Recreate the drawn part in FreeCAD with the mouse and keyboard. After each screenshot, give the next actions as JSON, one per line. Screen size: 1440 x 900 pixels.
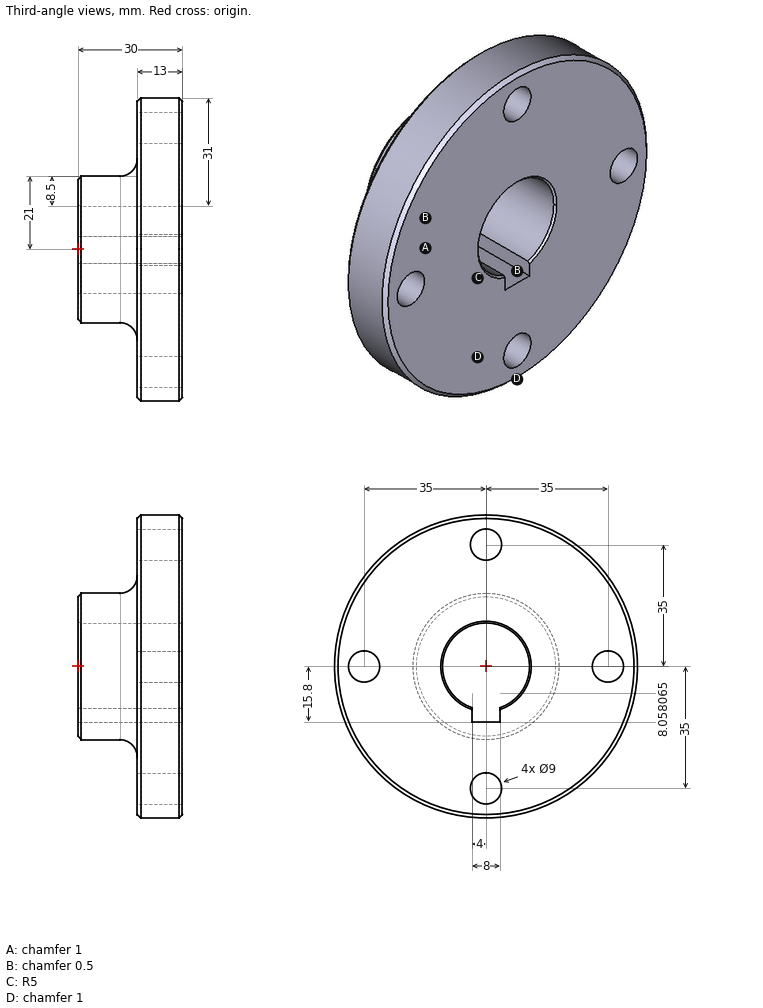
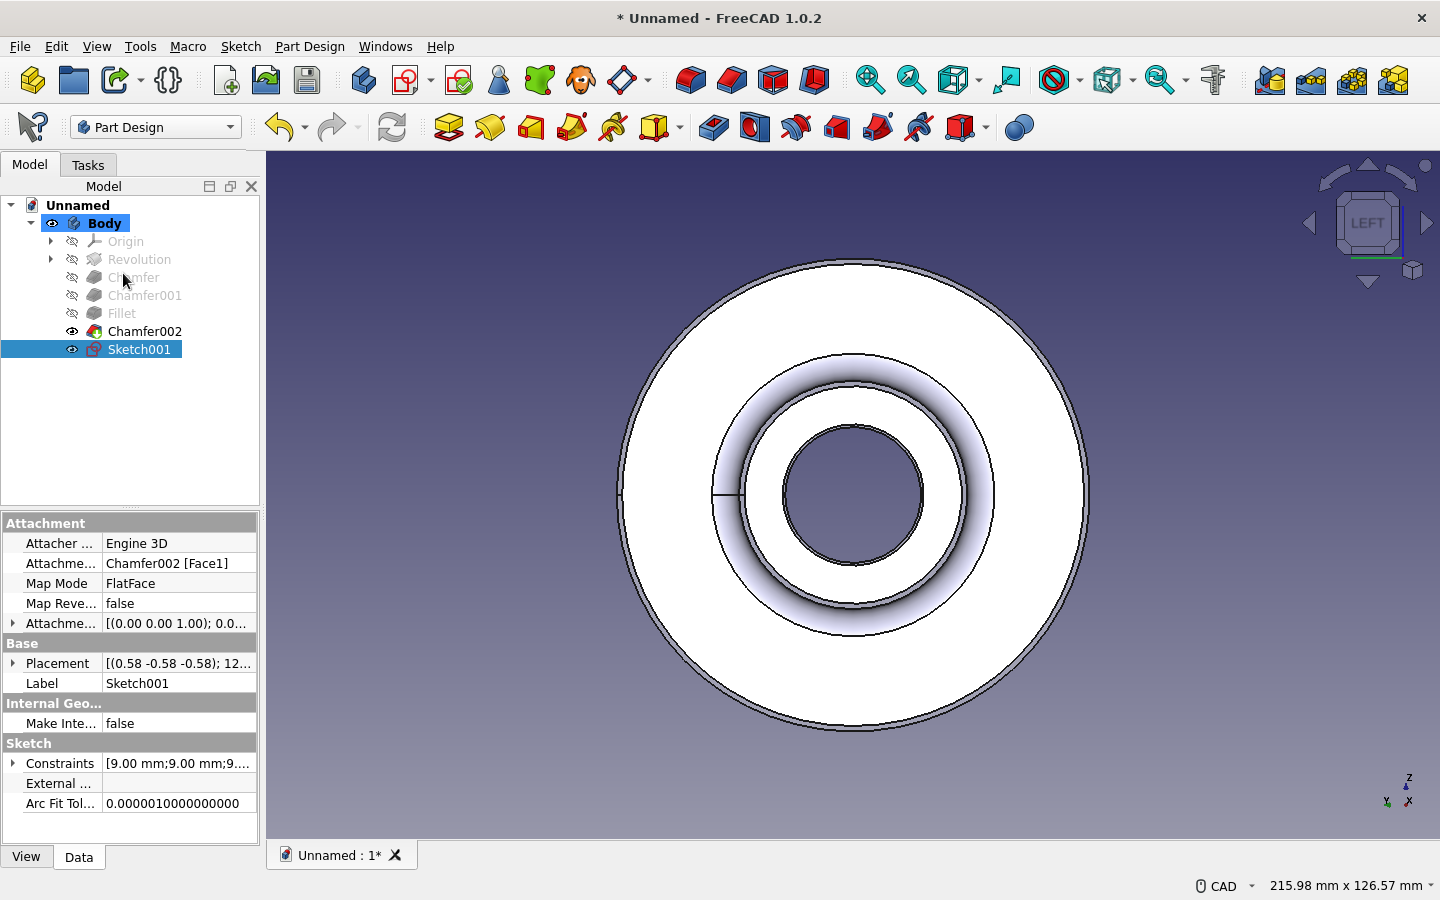
{"action": "left_click", "coordinate": [714, 128]}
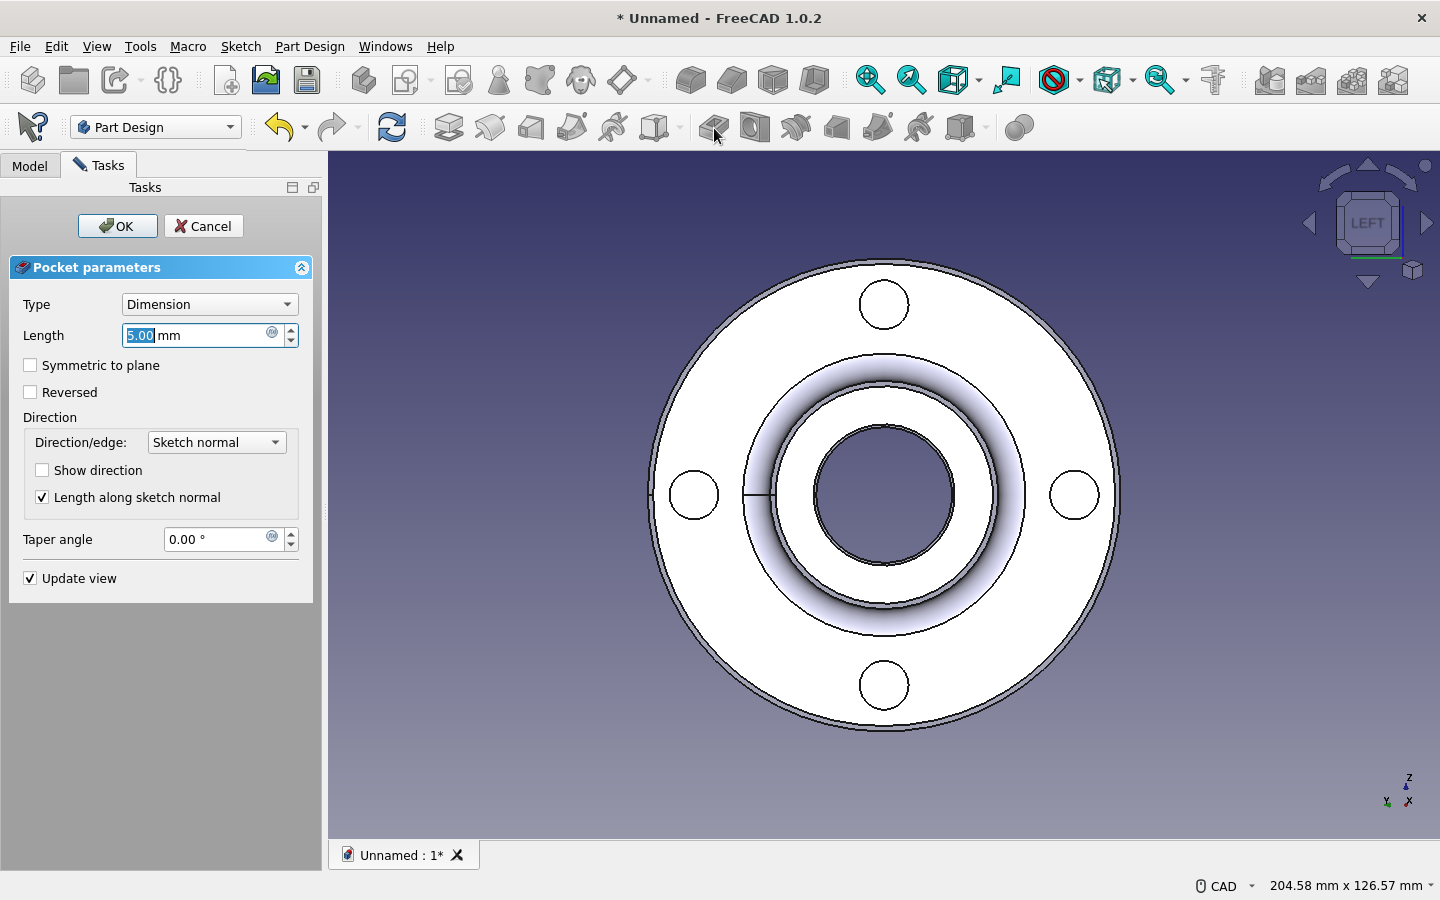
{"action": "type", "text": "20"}
{"action": "key", "text": "Tab"}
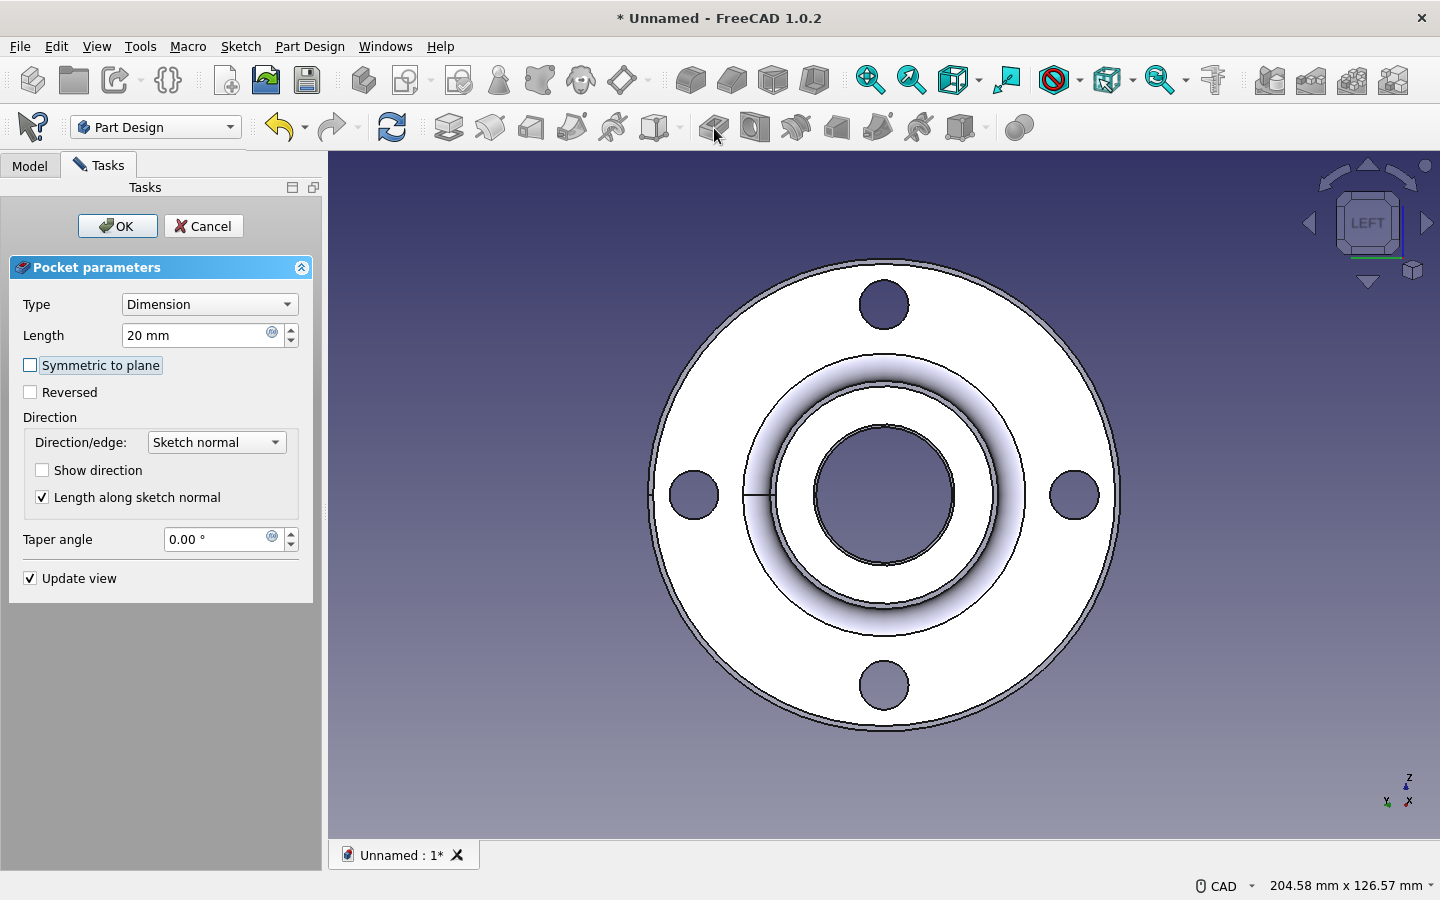
{"action": "left_click", "coordinate": [118, 226]}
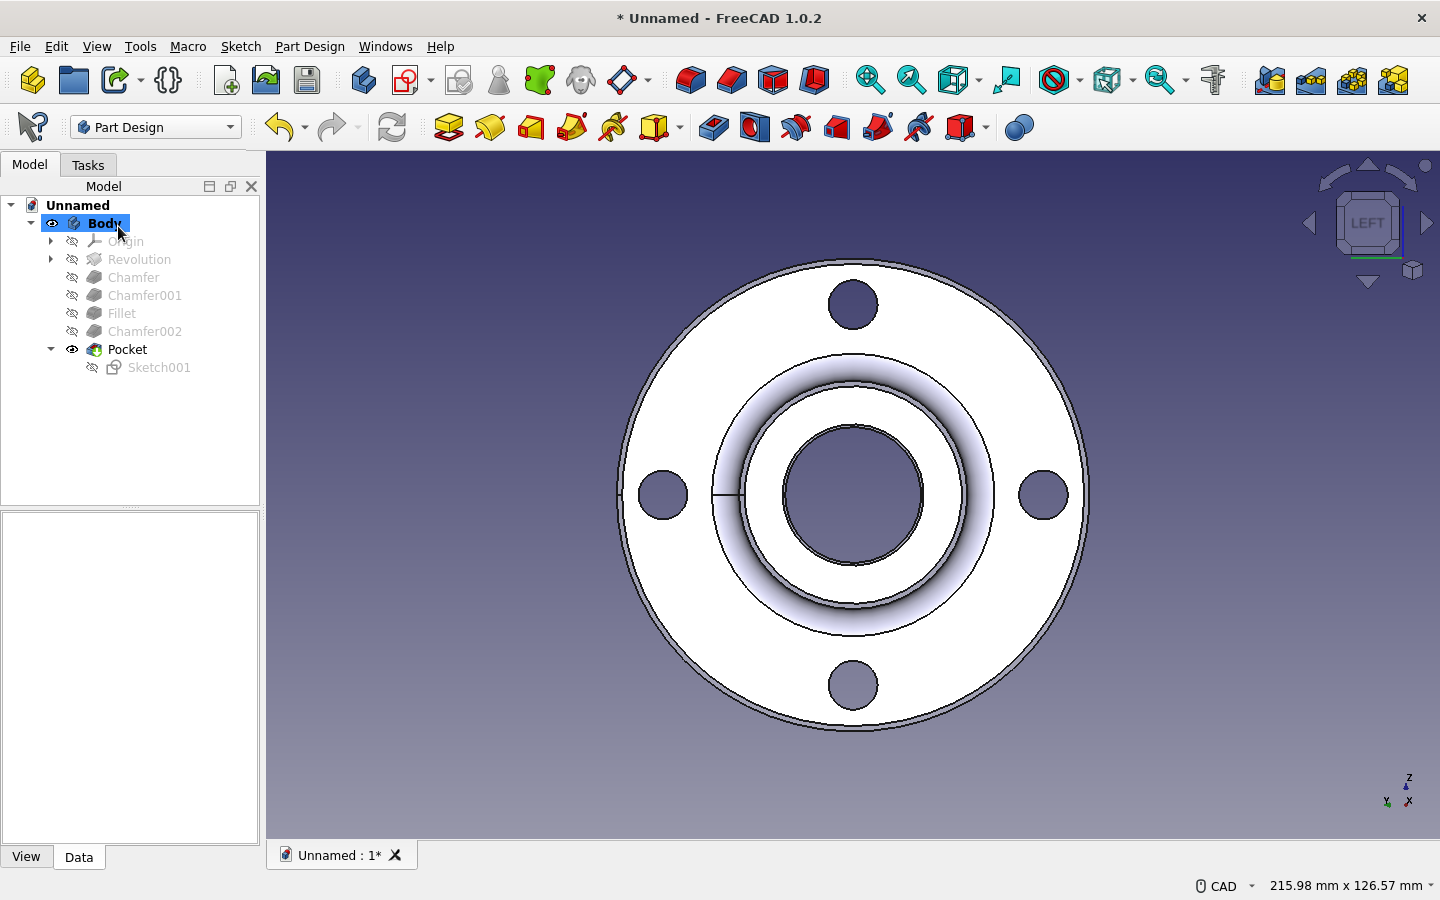
{"action": "key", "text": "0"}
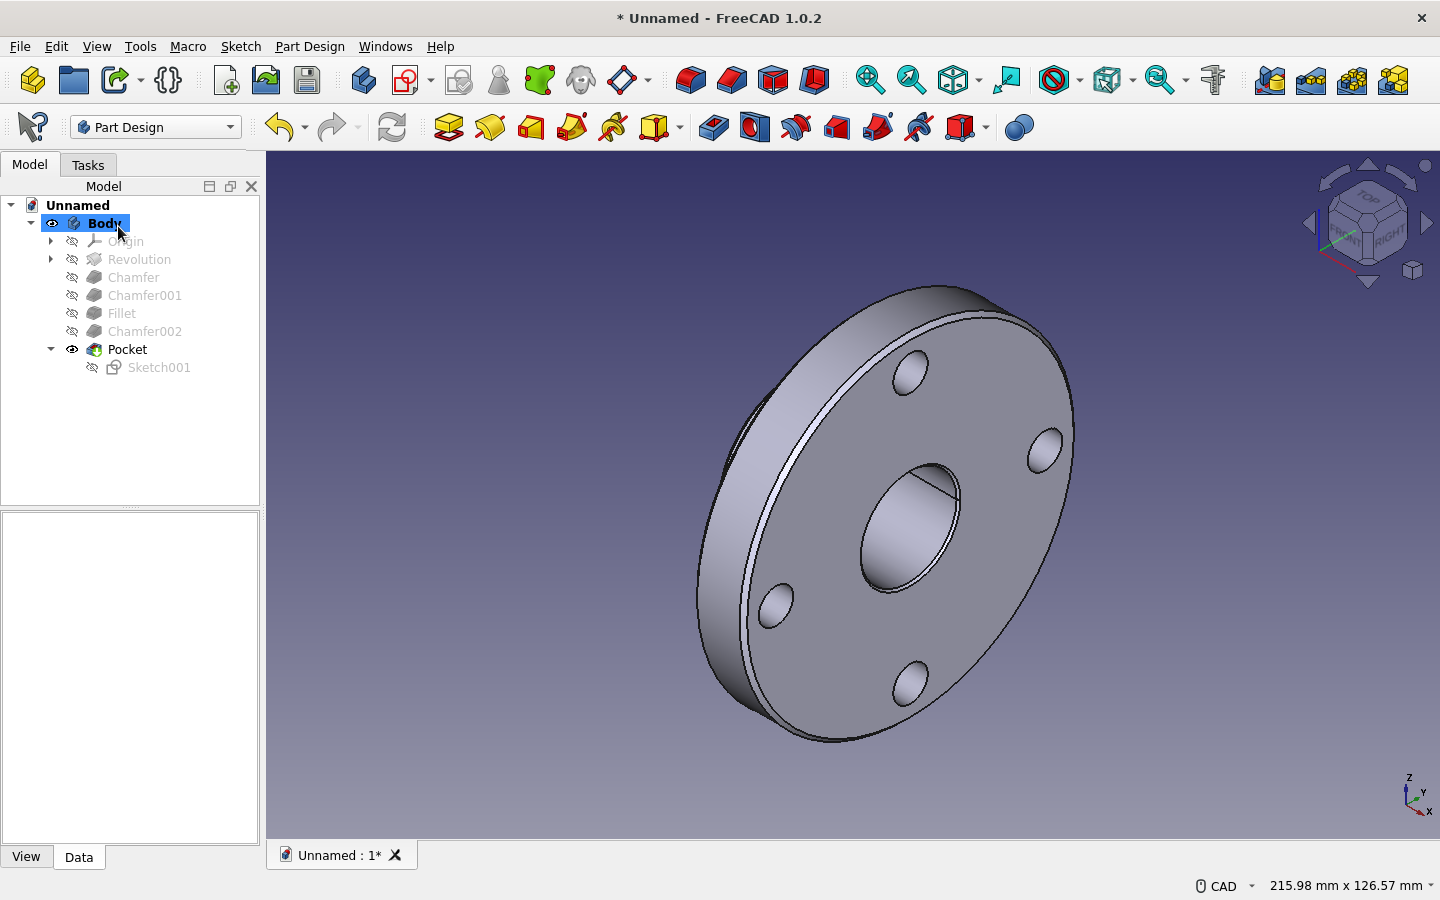
{"action": "left_click", "coordinate": [1004, 420]}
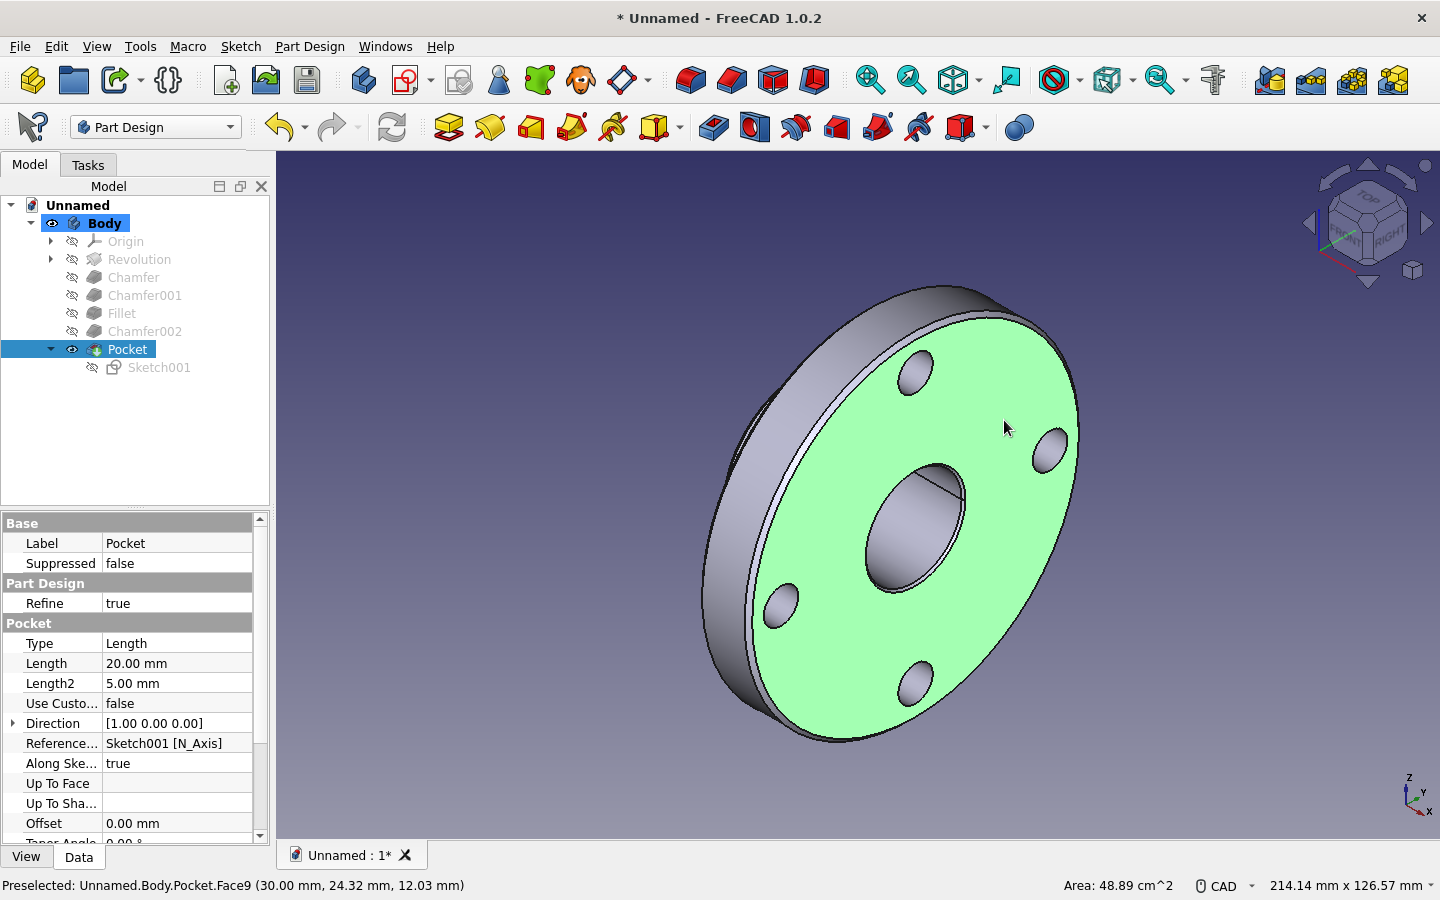
{"action": "left_click", "coordinate": [404, 80]}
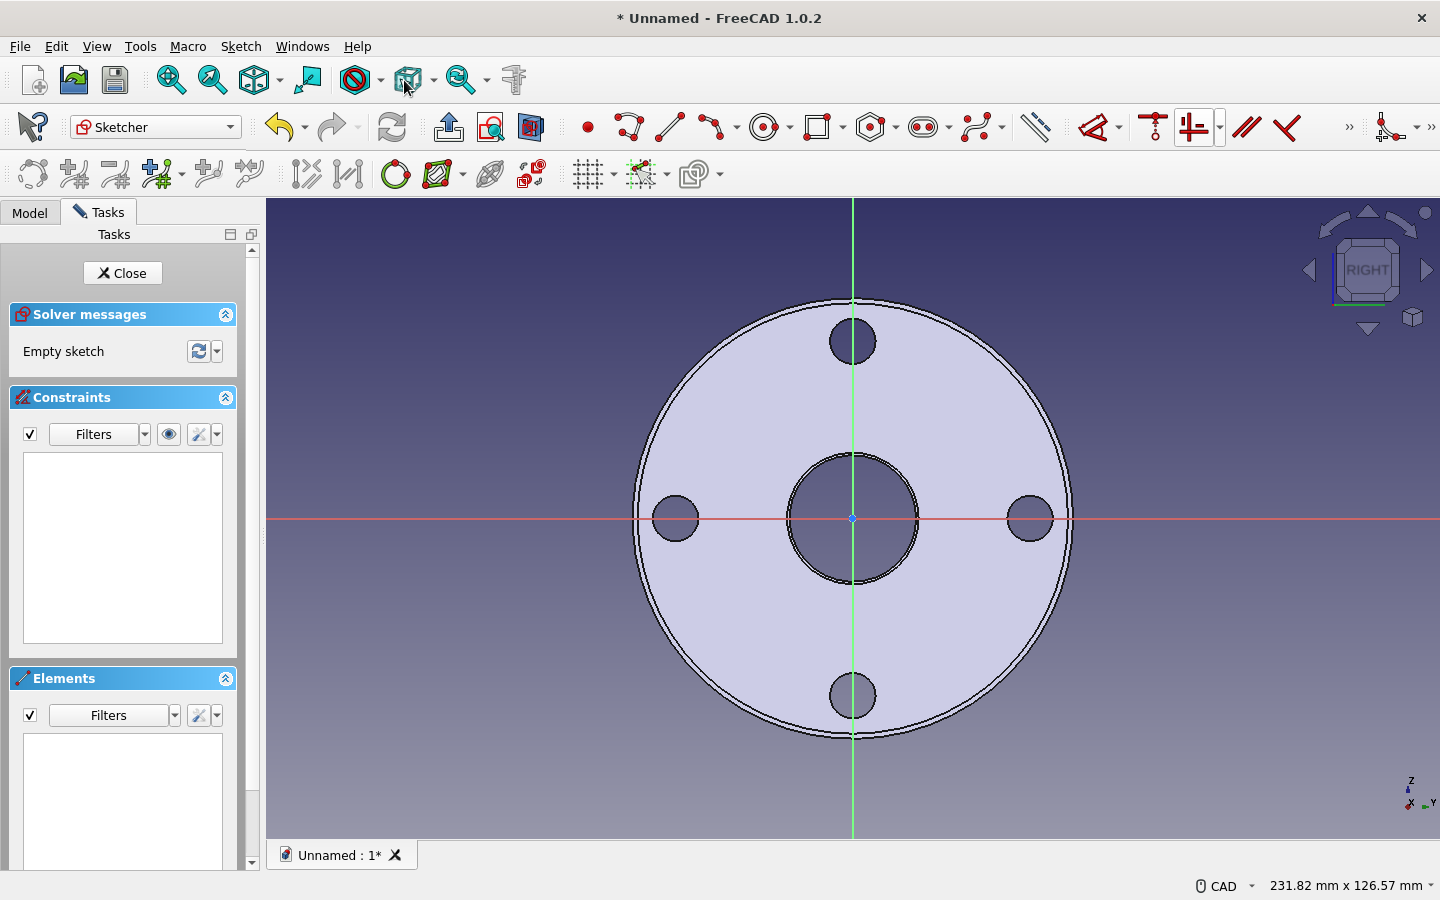
{"action": "scroll", "coordinate": [870, 569], "scroll_direction": "up", "scroll_amount": 8}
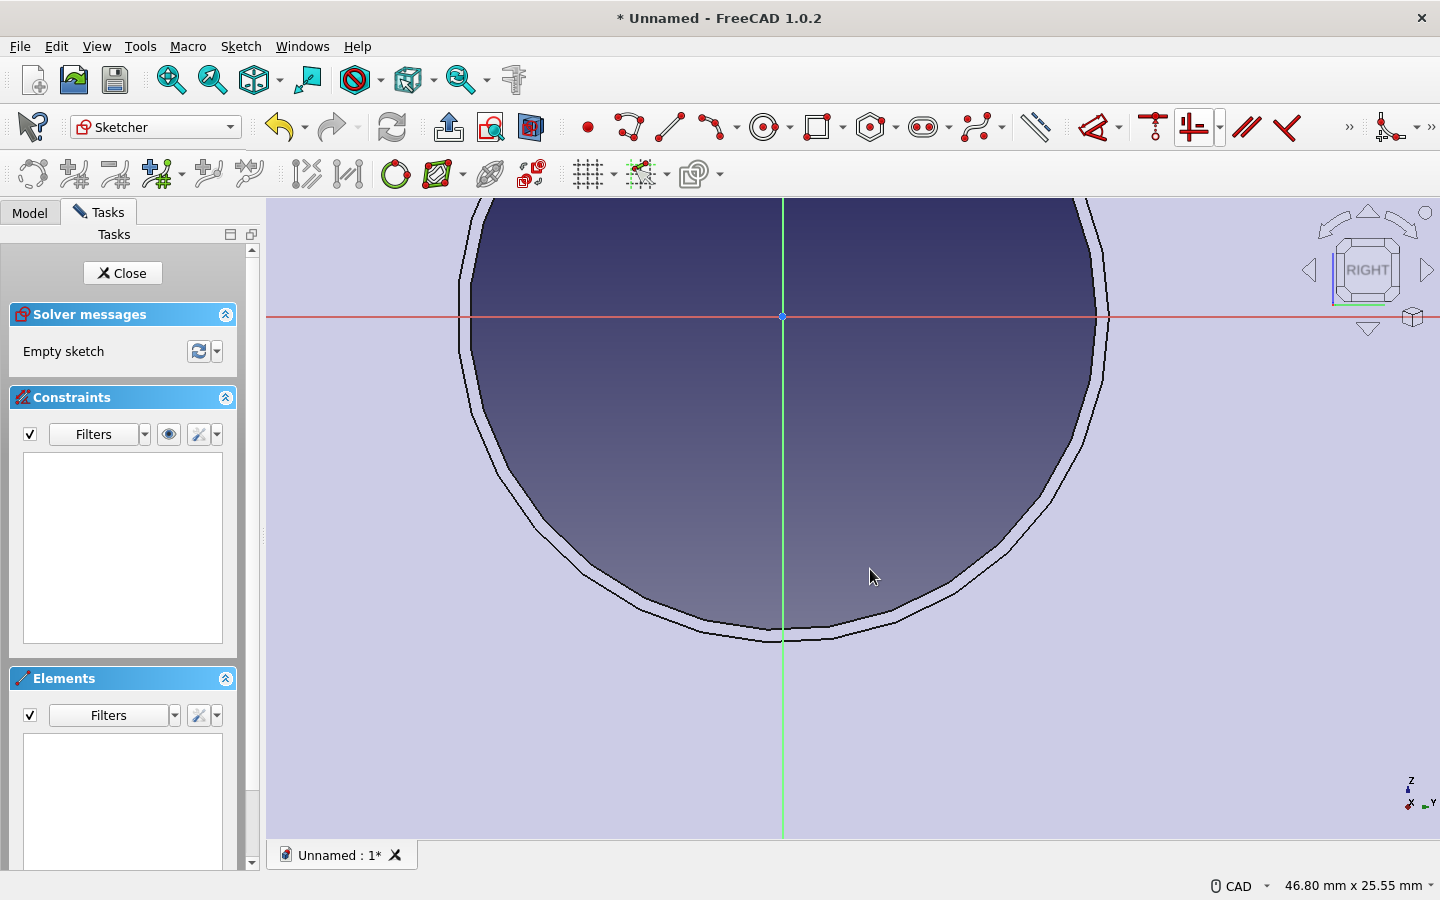
{"action": "left_click", "coordinate": [816, 128]}